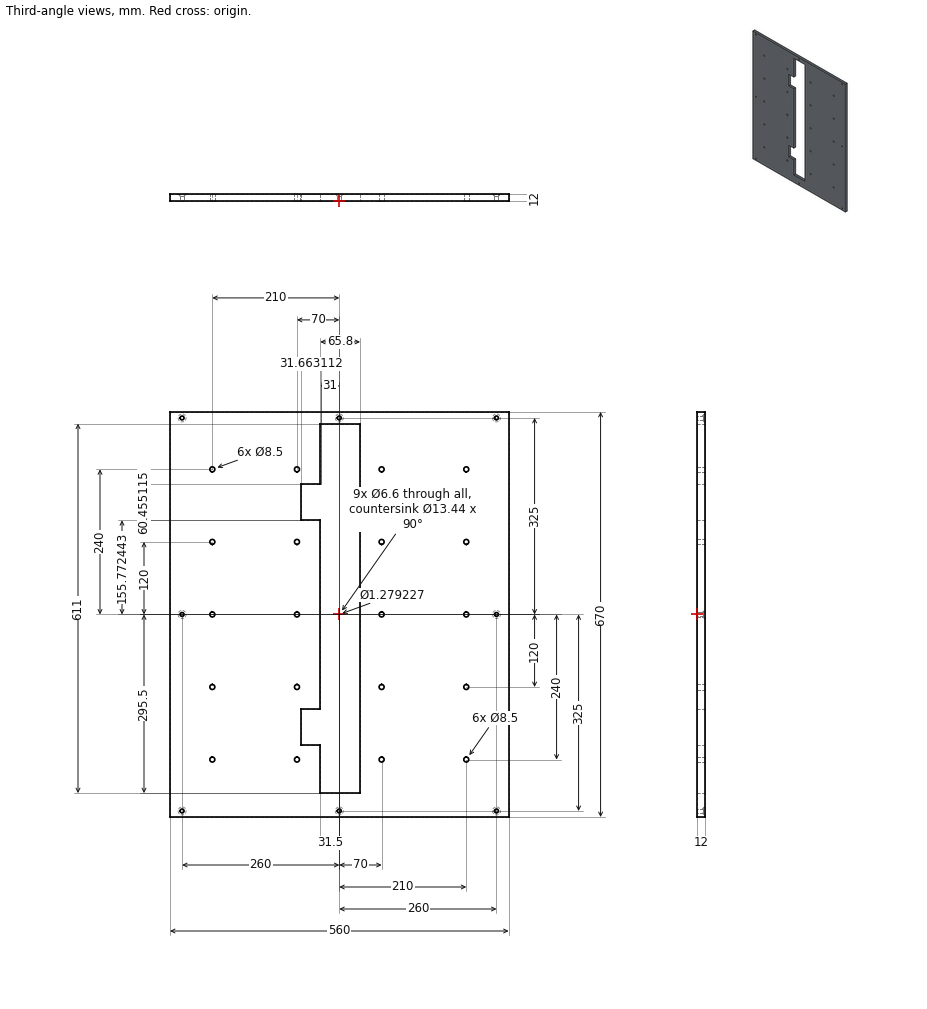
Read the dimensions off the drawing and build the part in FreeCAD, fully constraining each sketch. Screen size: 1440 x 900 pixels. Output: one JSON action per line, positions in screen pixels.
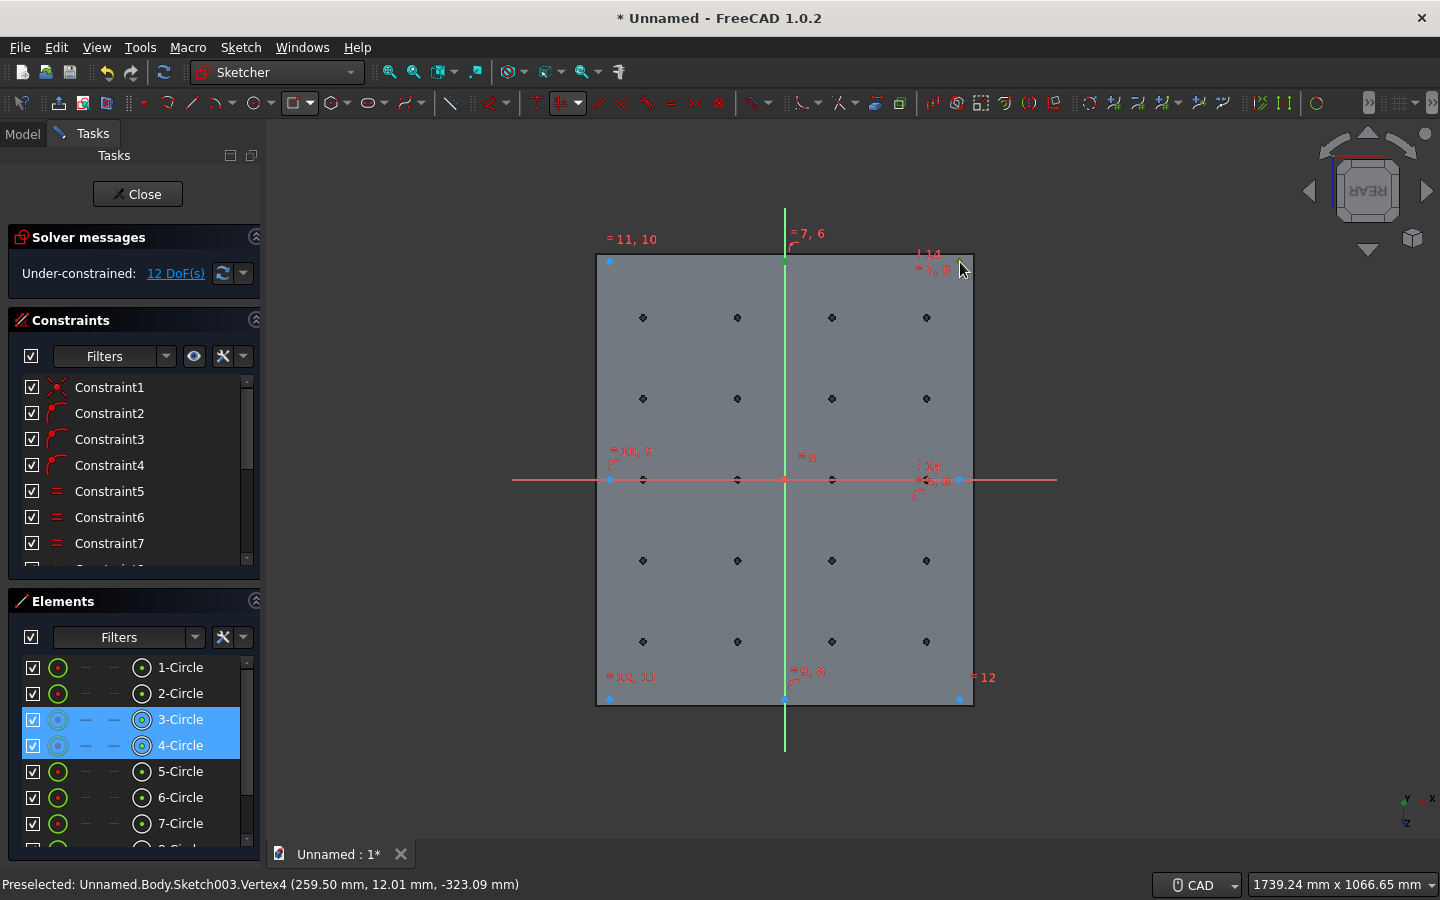
{"action": "key", "text": "h"}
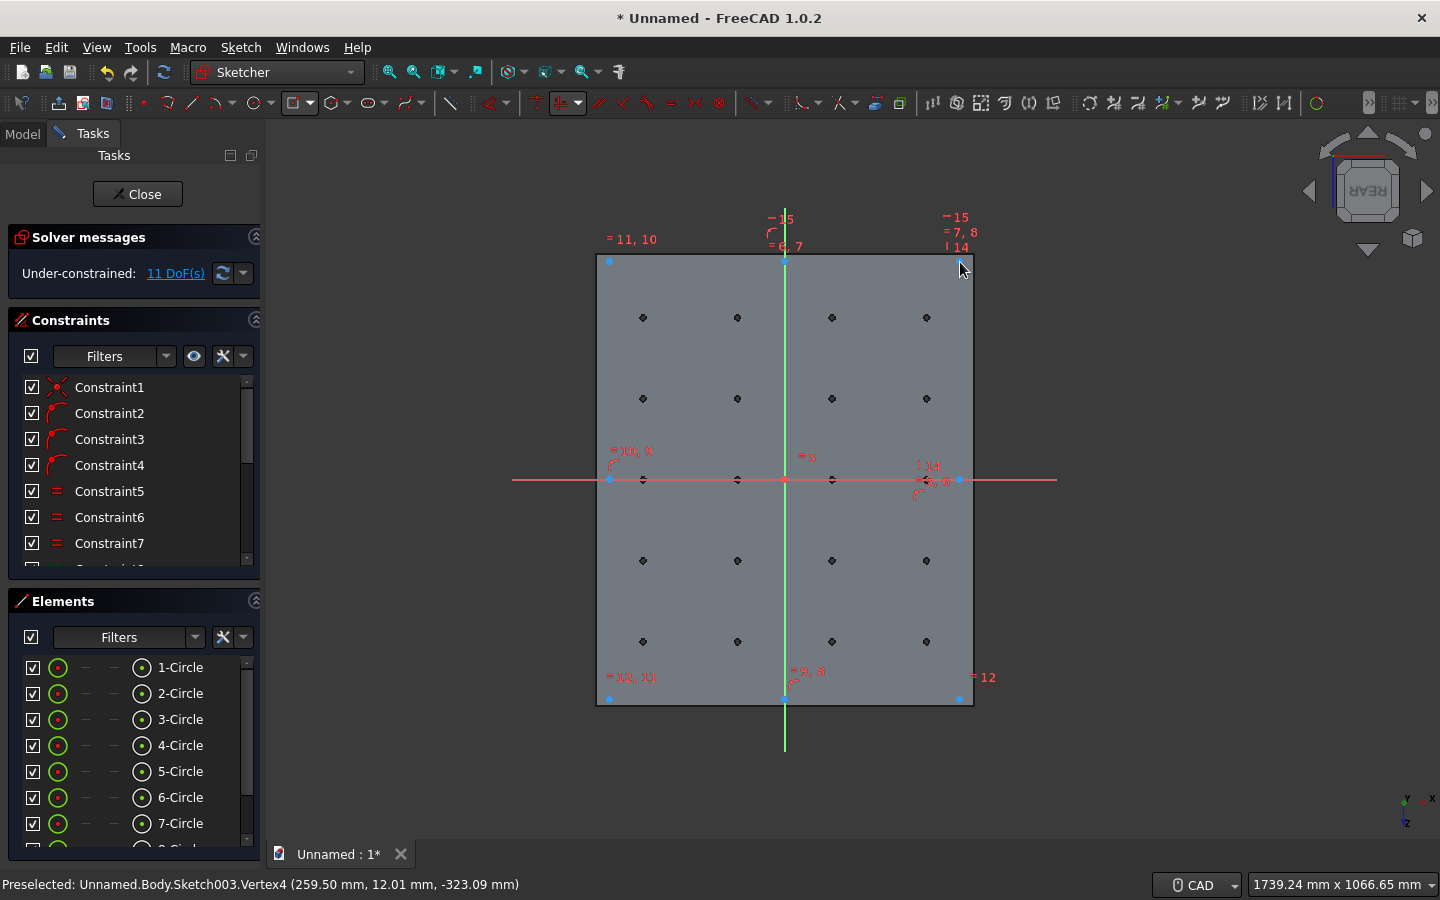
{"action": "left_click", "coordinate": [609, 480]}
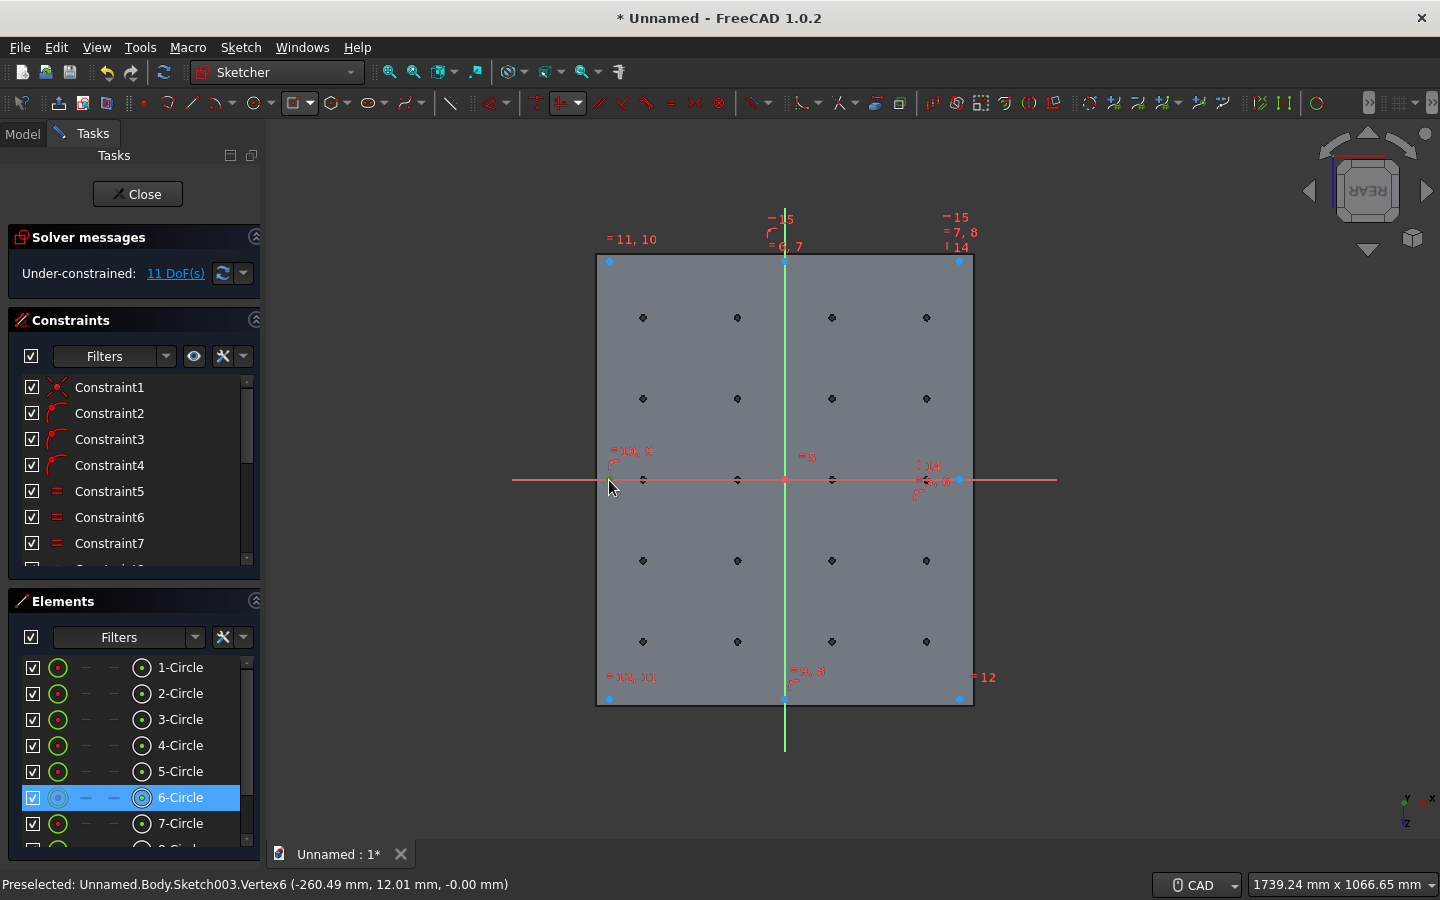
{"action": "left_click", "coordinate": [609, 262]}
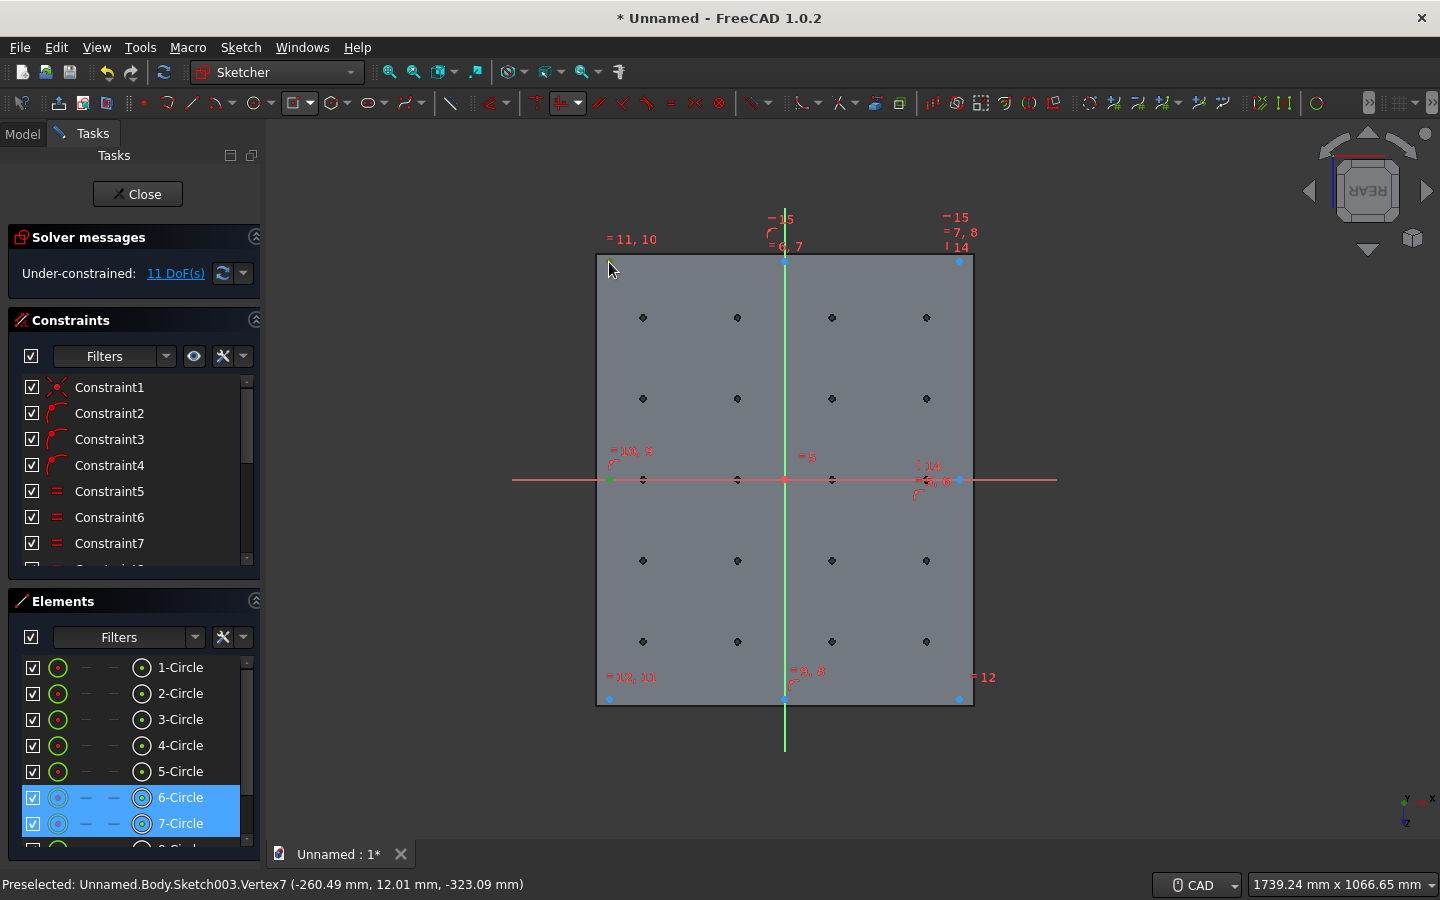
{"action": "left_click", "coordinate": [580, 104]}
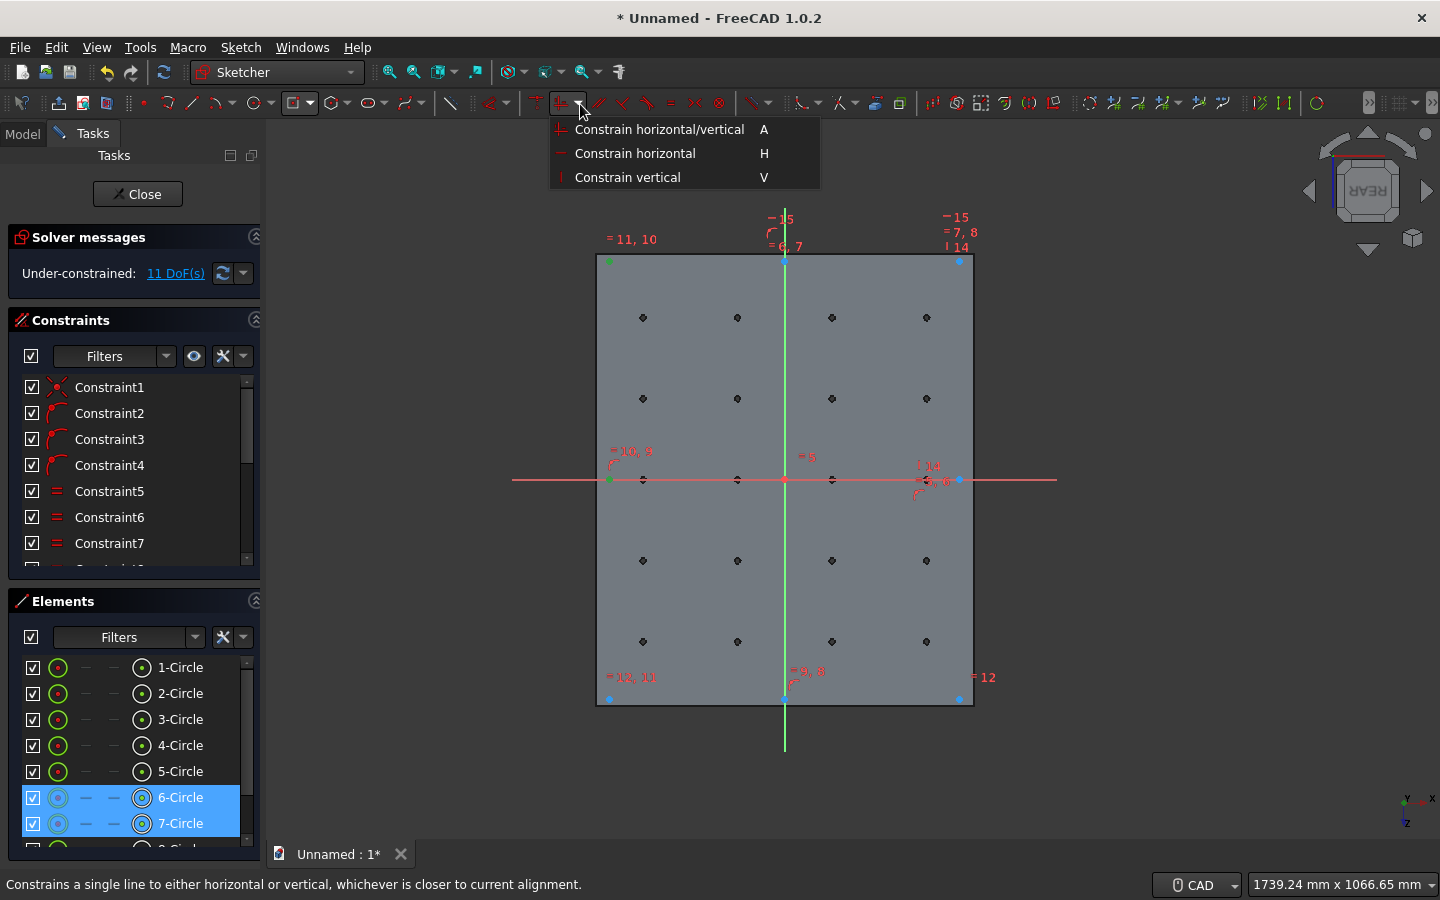
{"action": "left_click", "coordinate": [685, 177]}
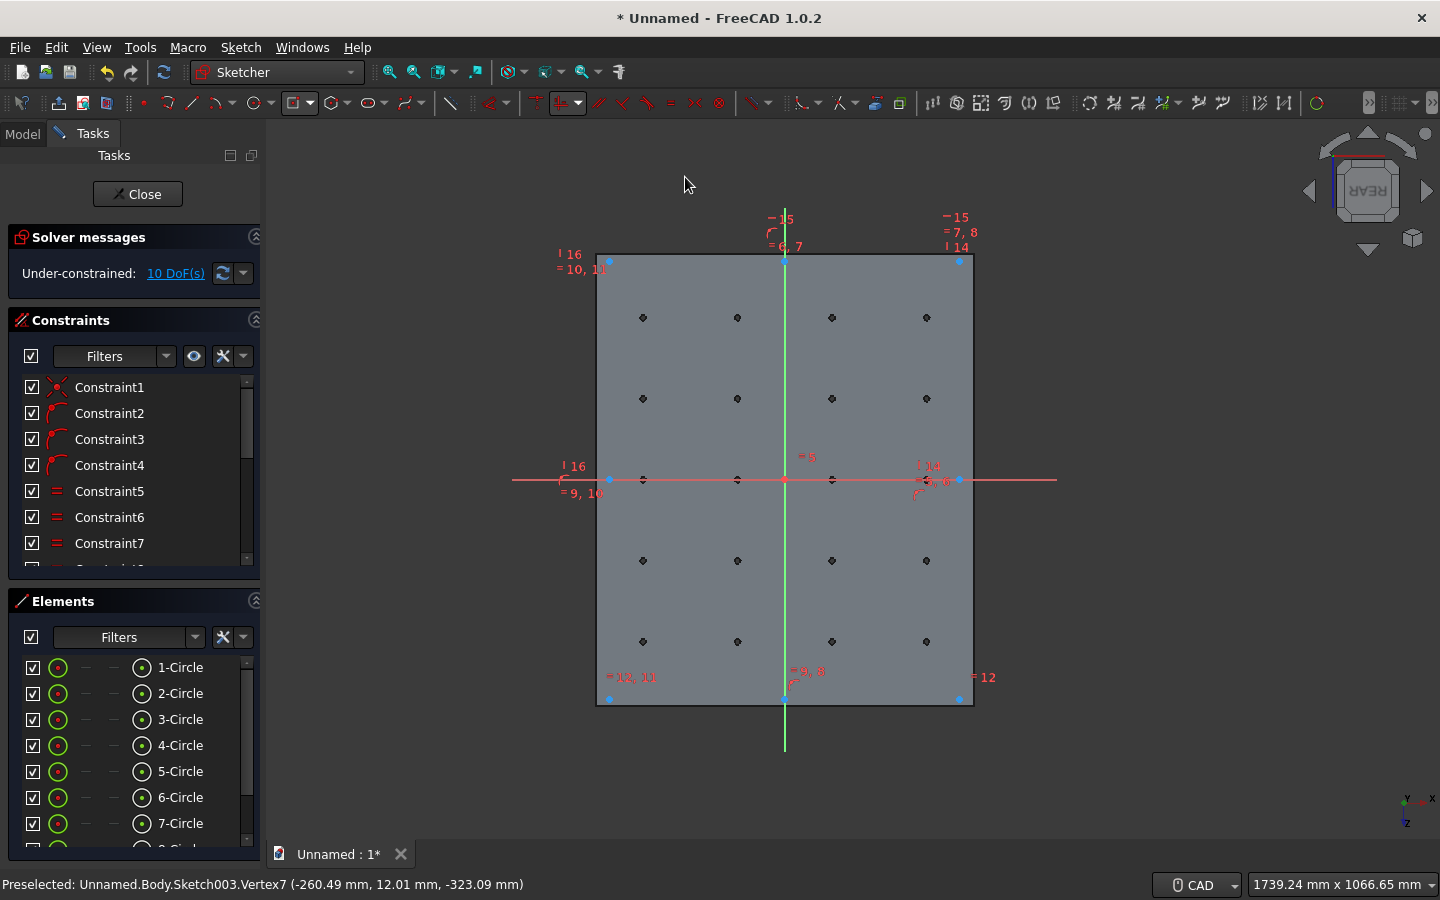
{"action": "left_click", "coordinate": [785, 262]}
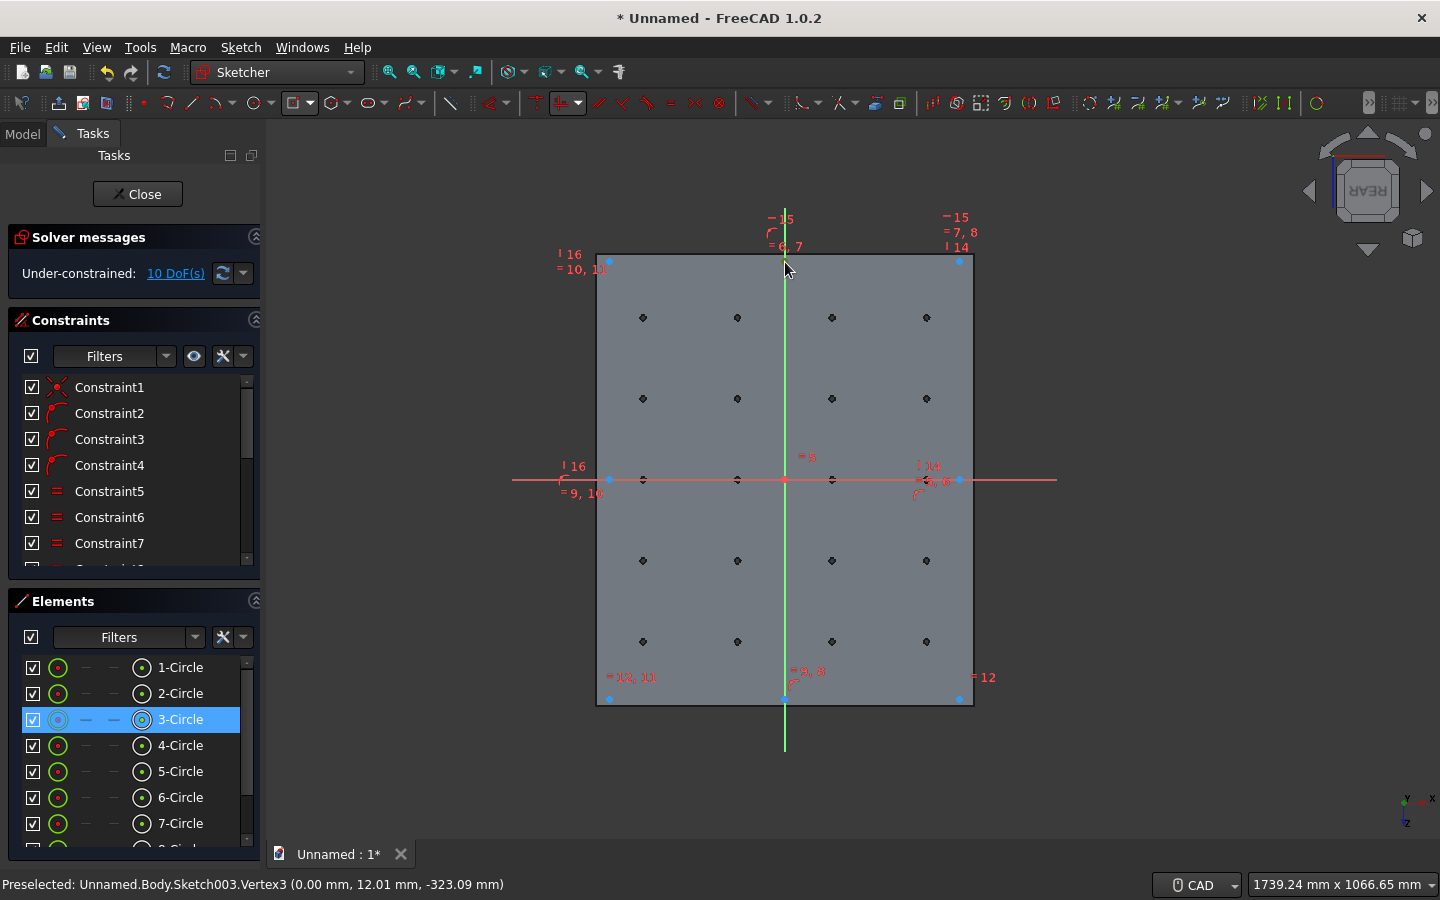
{"action": "left_click", "coordinate": [609, 262]}